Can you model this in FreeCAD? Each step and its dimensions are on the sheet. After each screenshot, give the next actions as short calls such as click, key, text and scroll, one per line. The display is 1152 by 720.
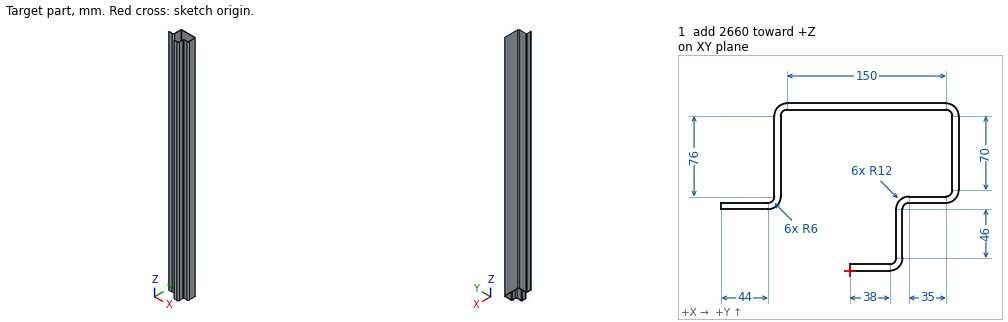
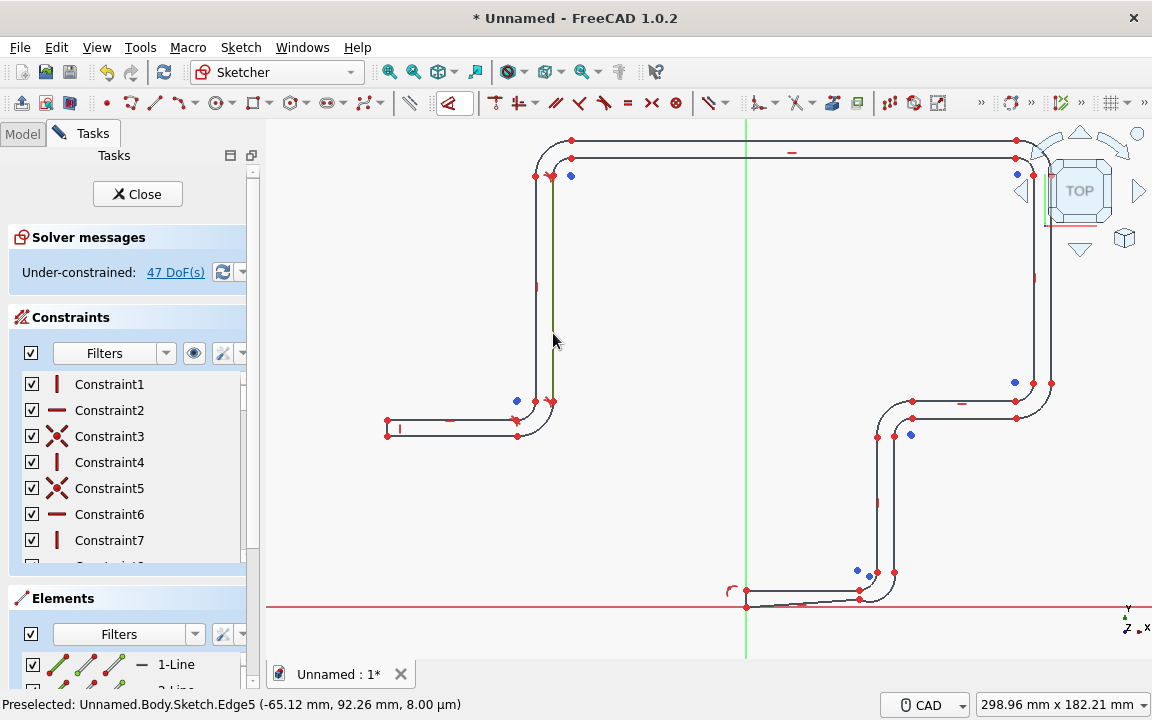
click(534, 432)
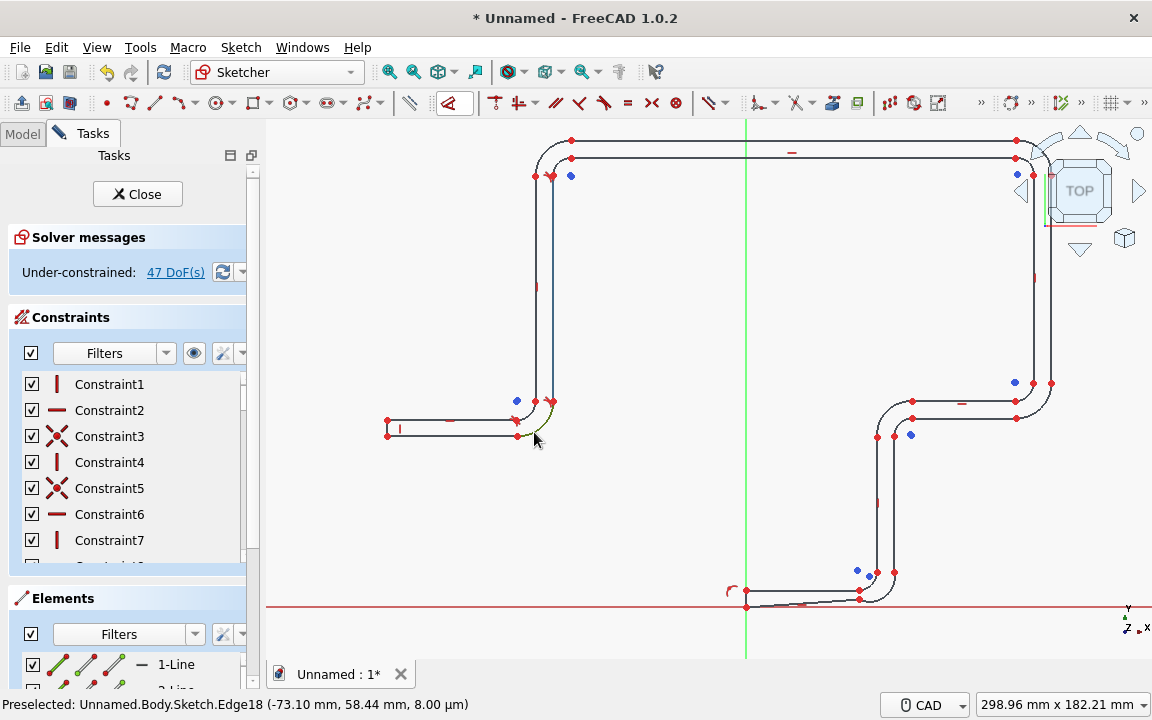
key(t)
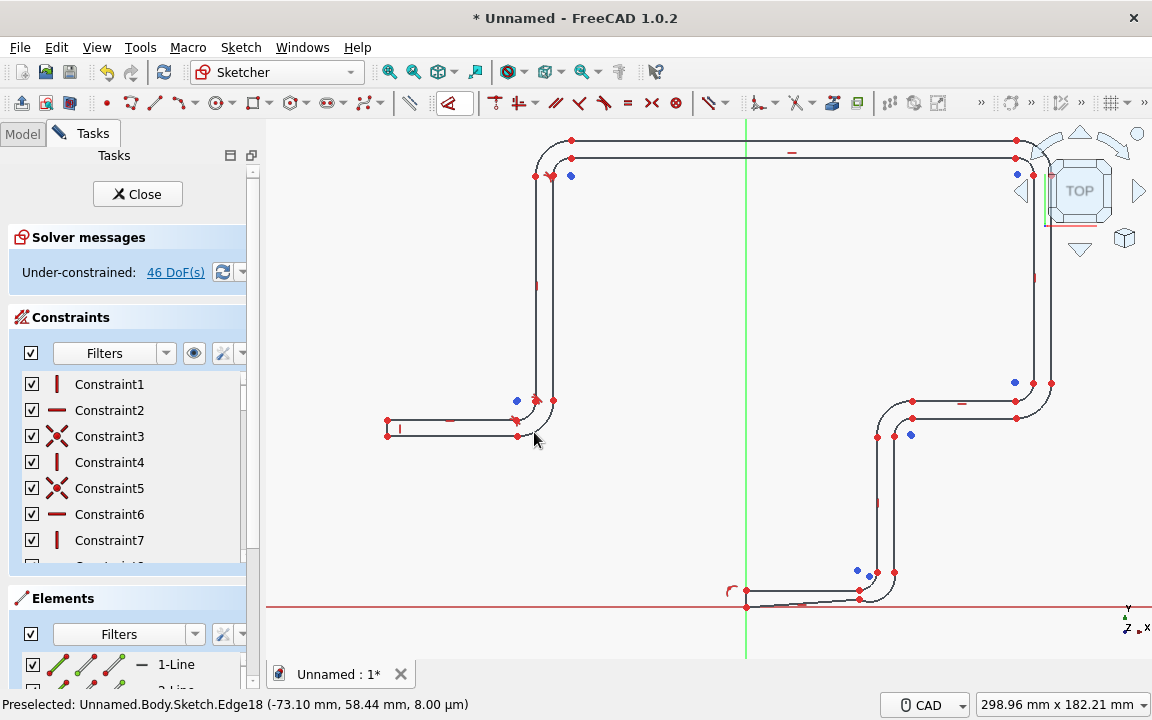
click(553, 333)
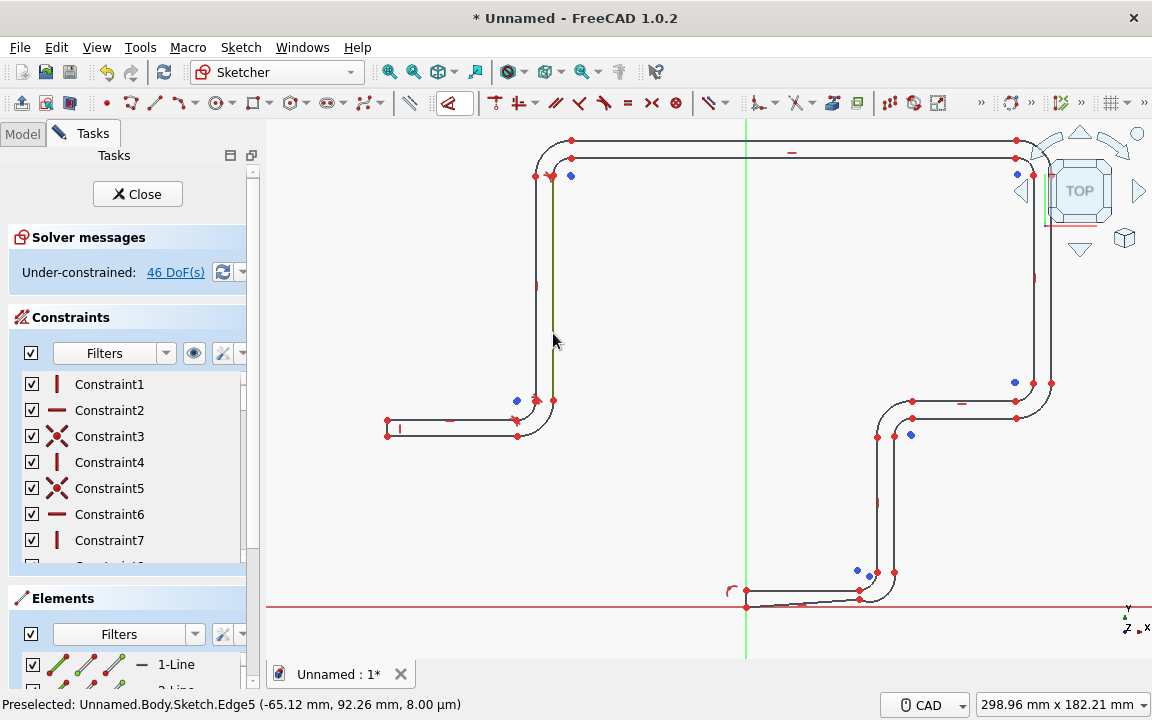
click(559, 163)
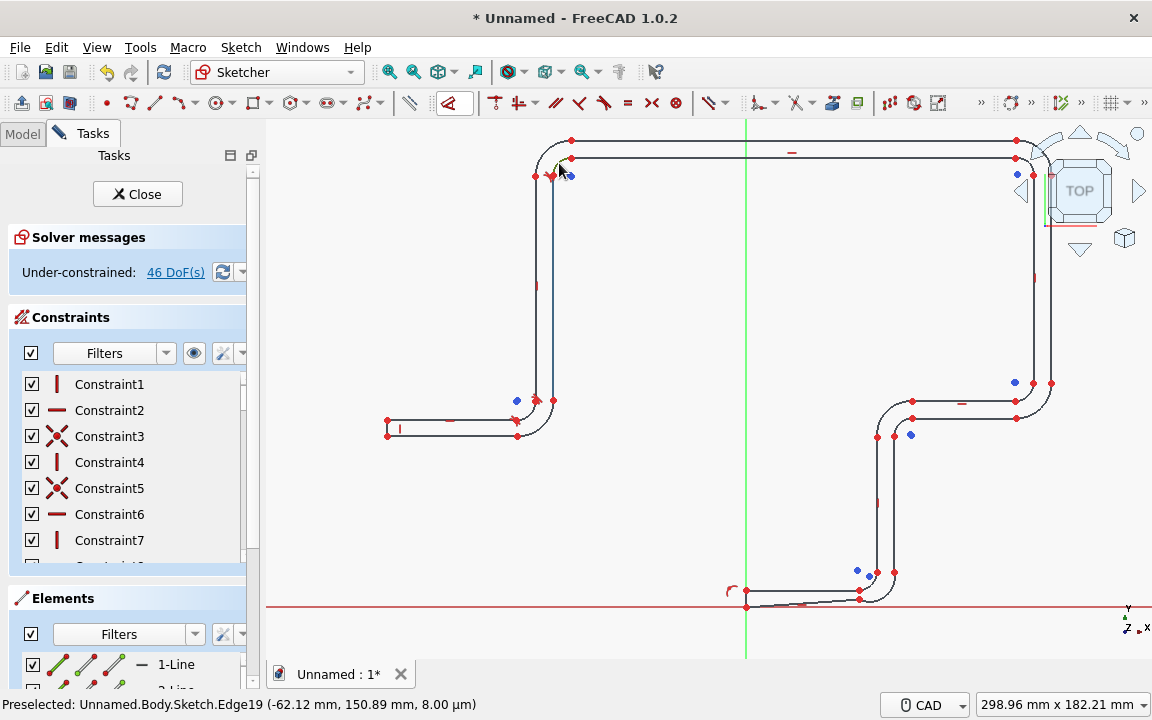
key(t)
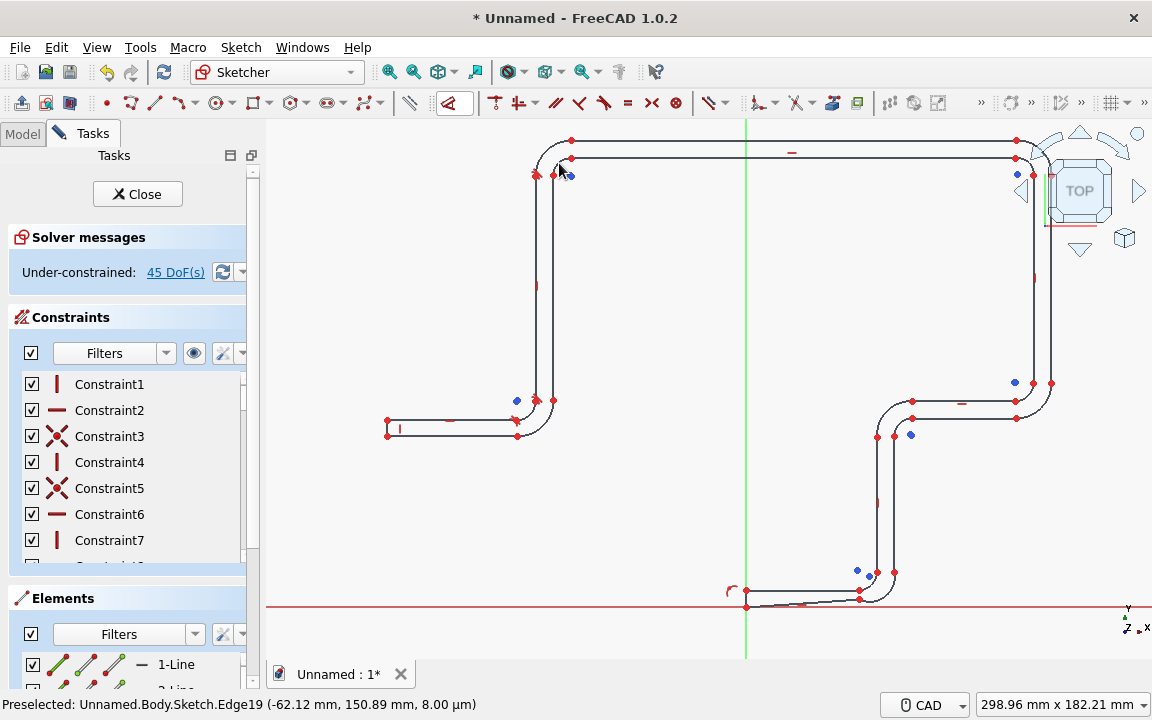
click(705, 158)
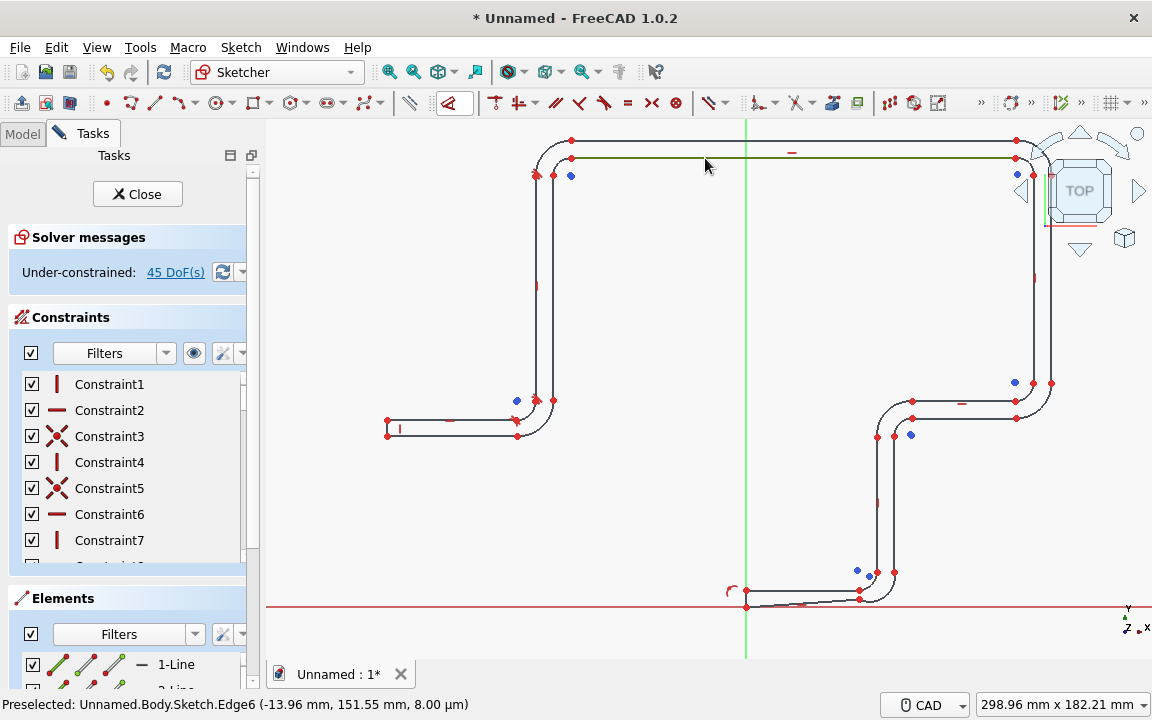
click(559, 163)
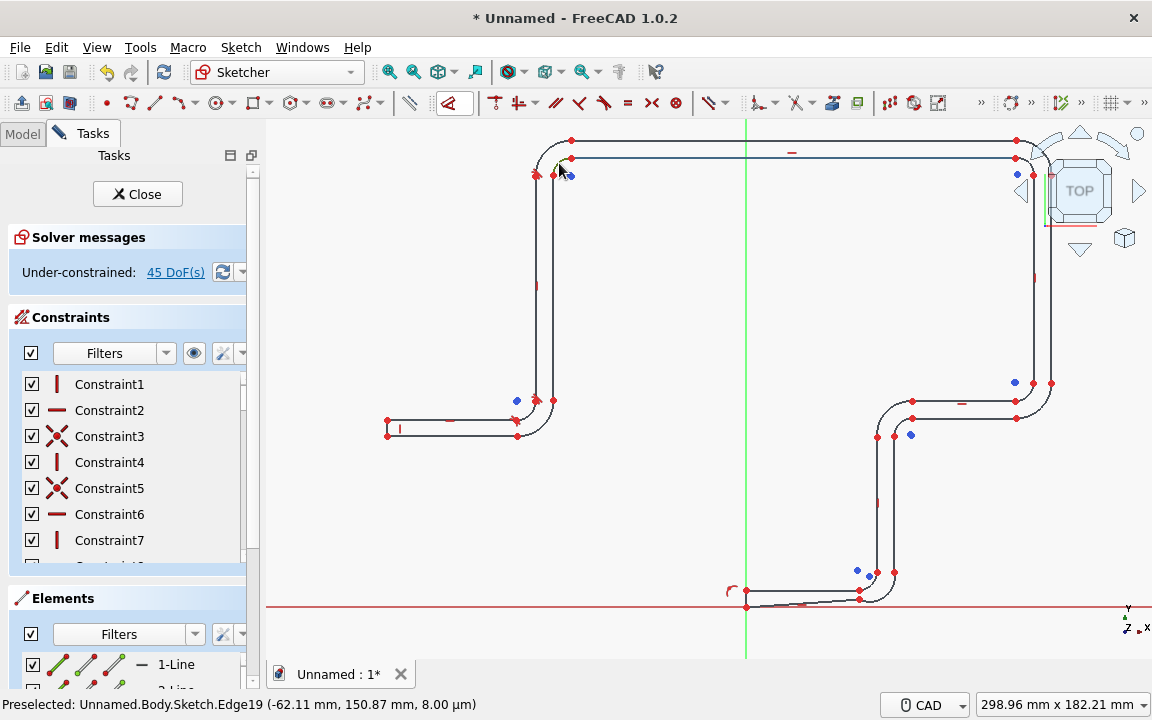
key(t)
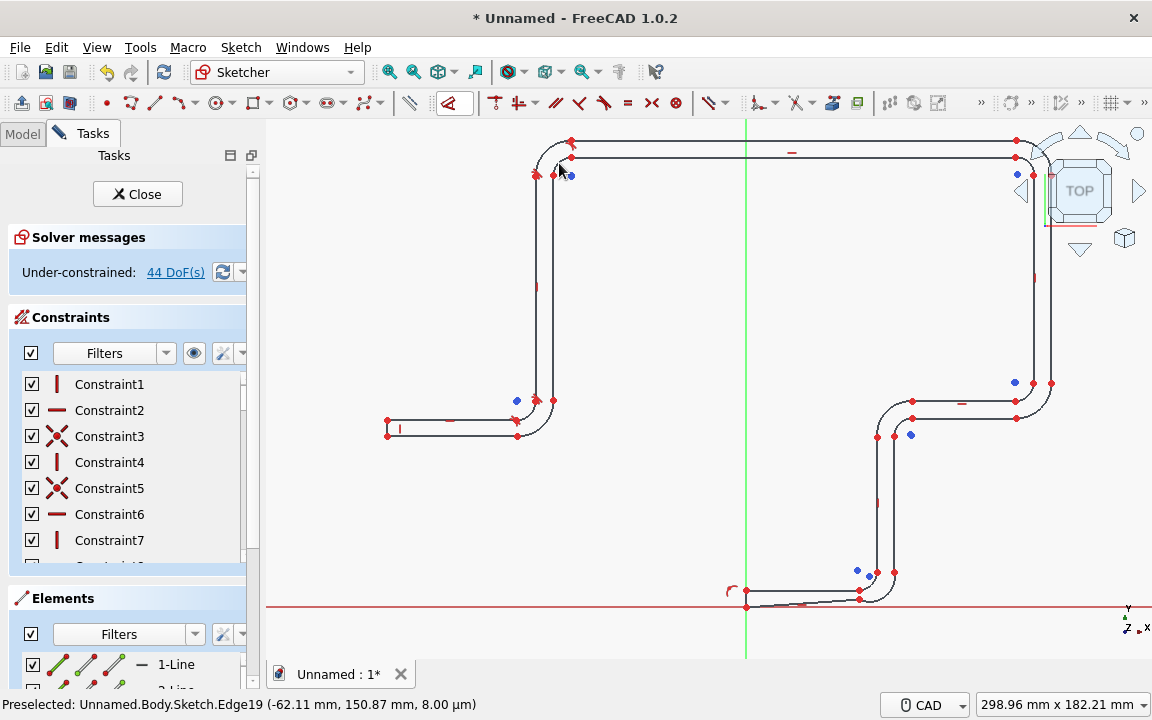
click(705, 158)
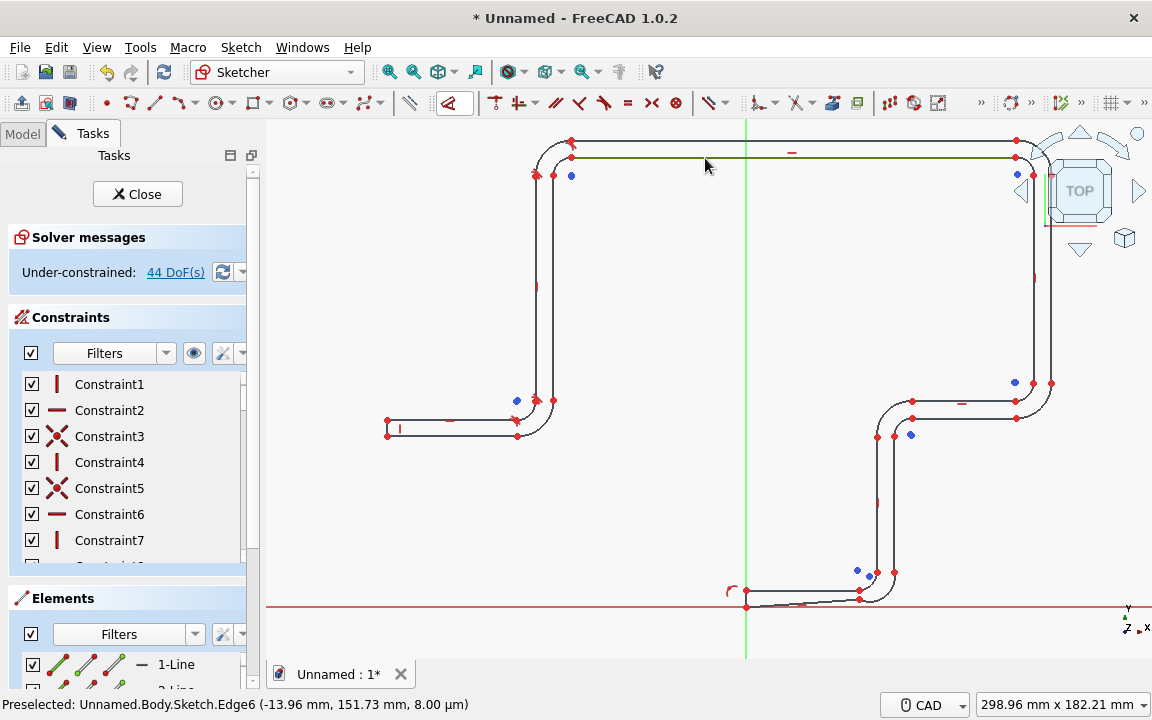
scroll(479, 421, down, 2)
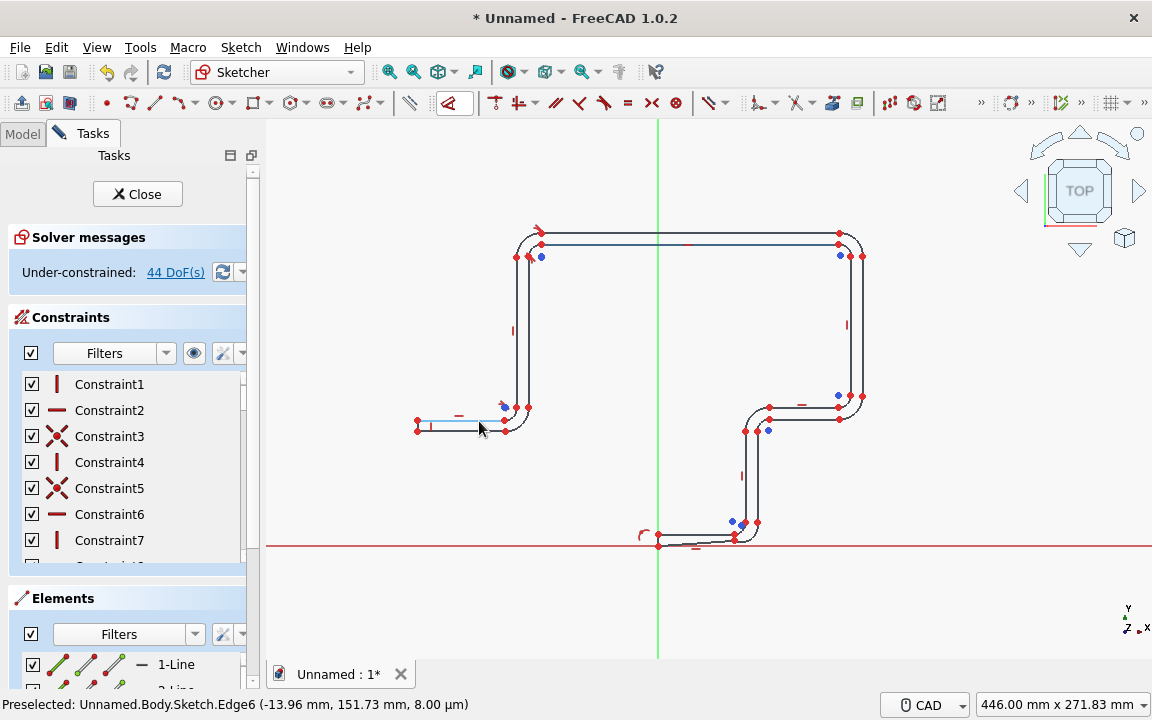
scroll(848, 248, up, 2)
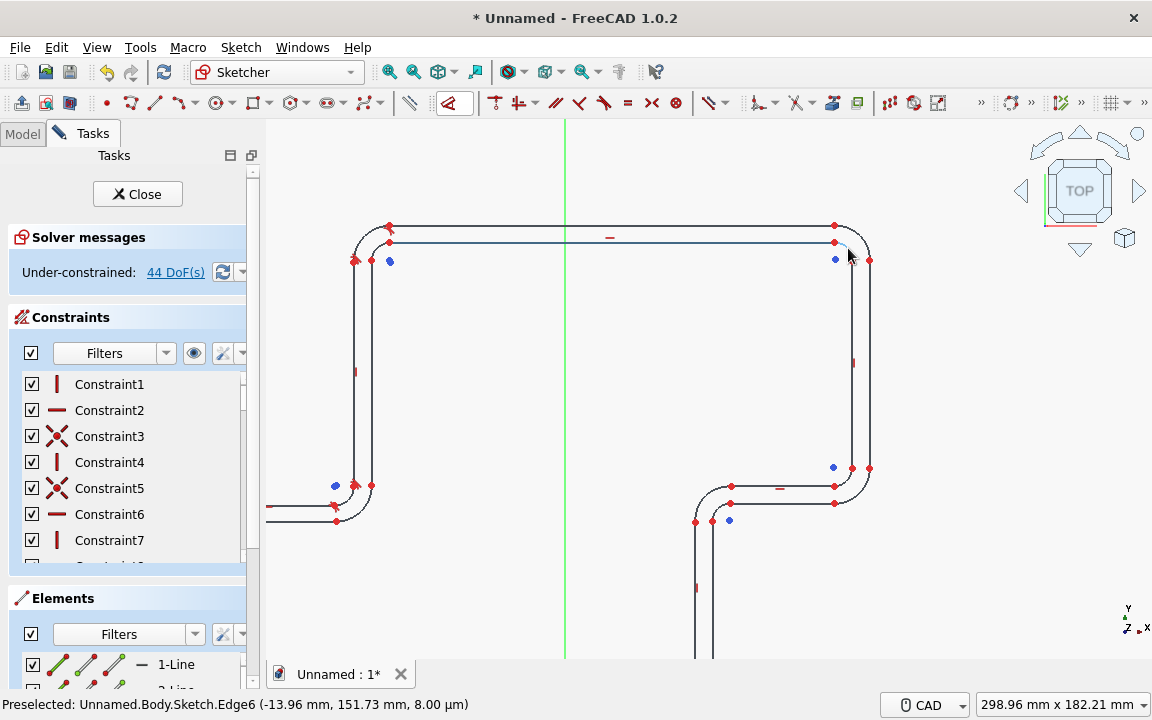
click(847, 248)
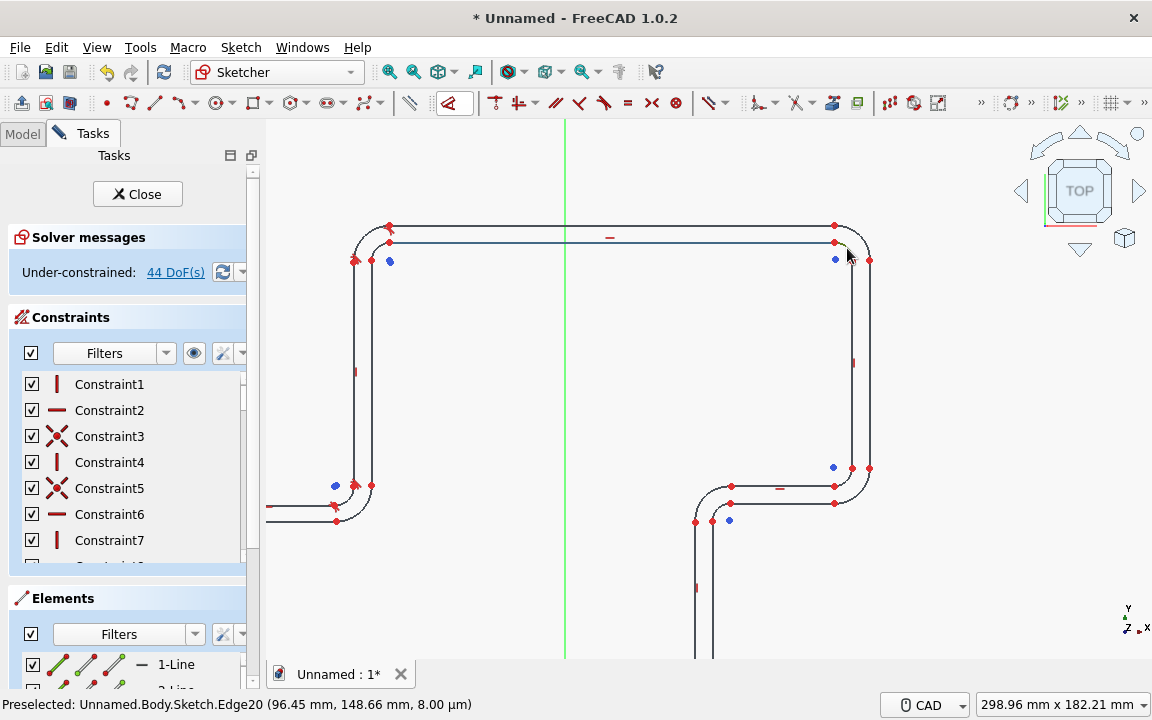
click(604, 104)